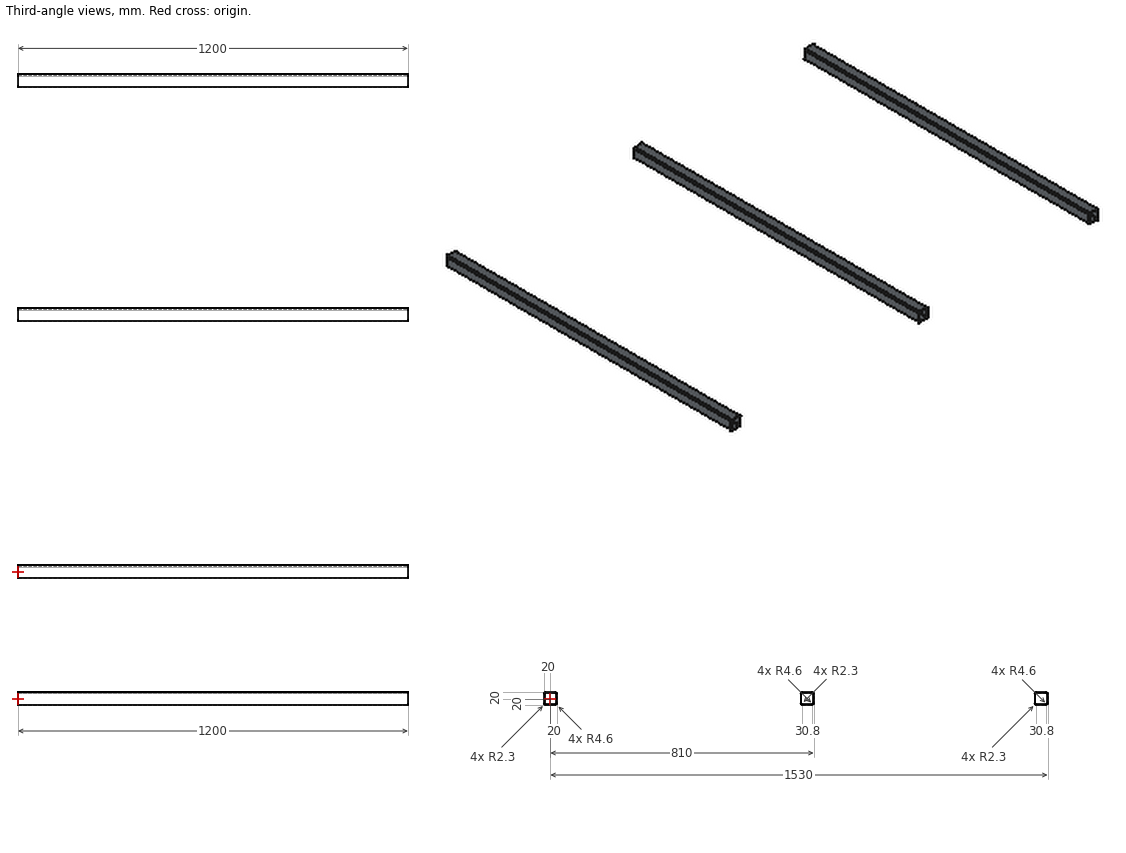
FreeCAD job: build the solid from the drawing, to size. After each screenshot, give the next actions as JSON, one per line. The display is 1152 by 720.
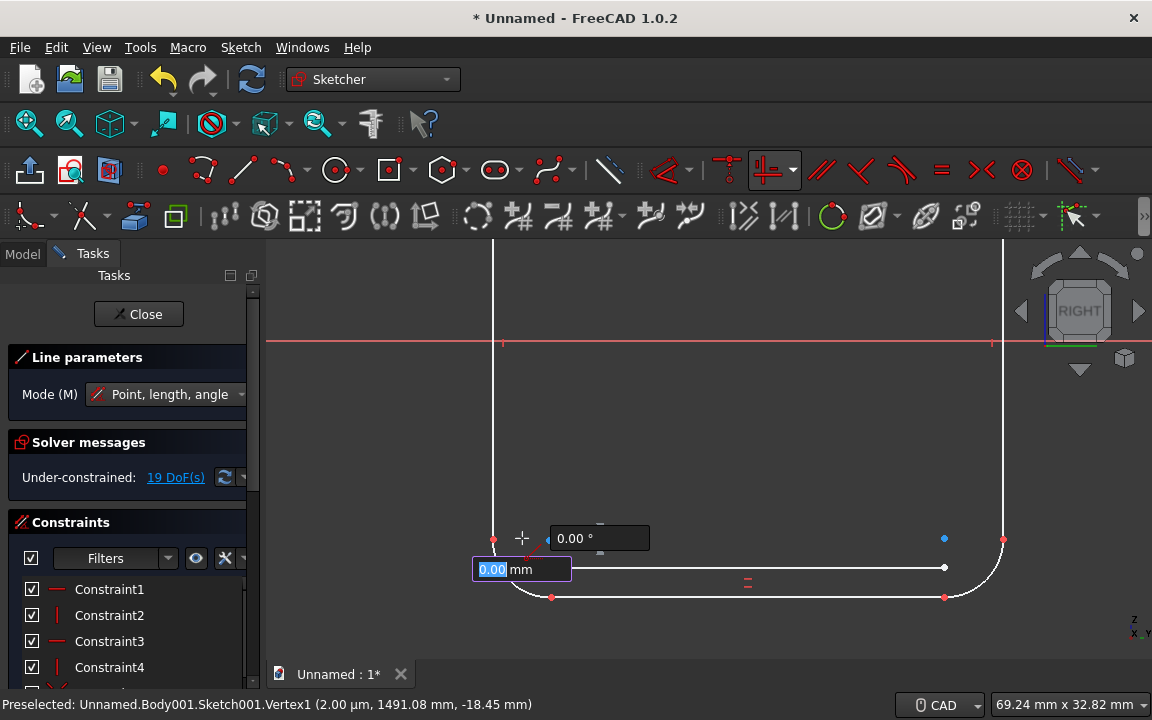
{"action": "scroll", "coordinate": [510, 581], "scroll_direction": "down", "scroll_amount": 3}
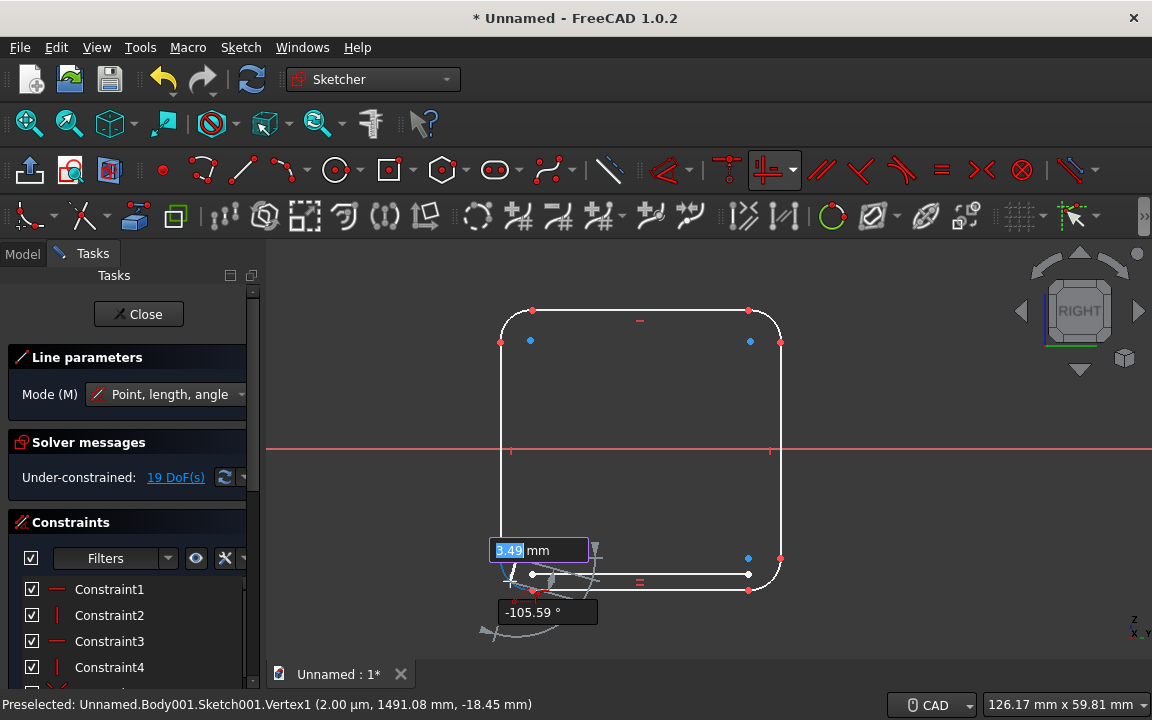
{"action": "left_click", "coordinate": [517, 341]}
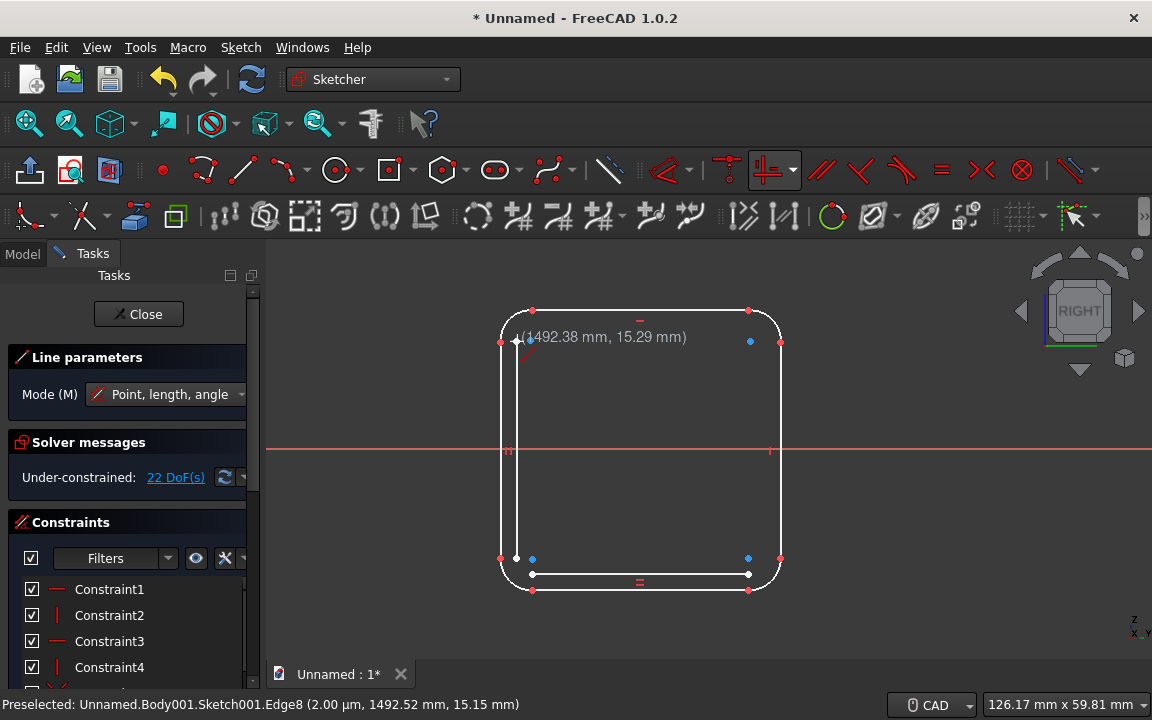
{"action": "left_click", "coordinate": [533, 325]}
{"action": "left_click", "coordinate": [749, 325]}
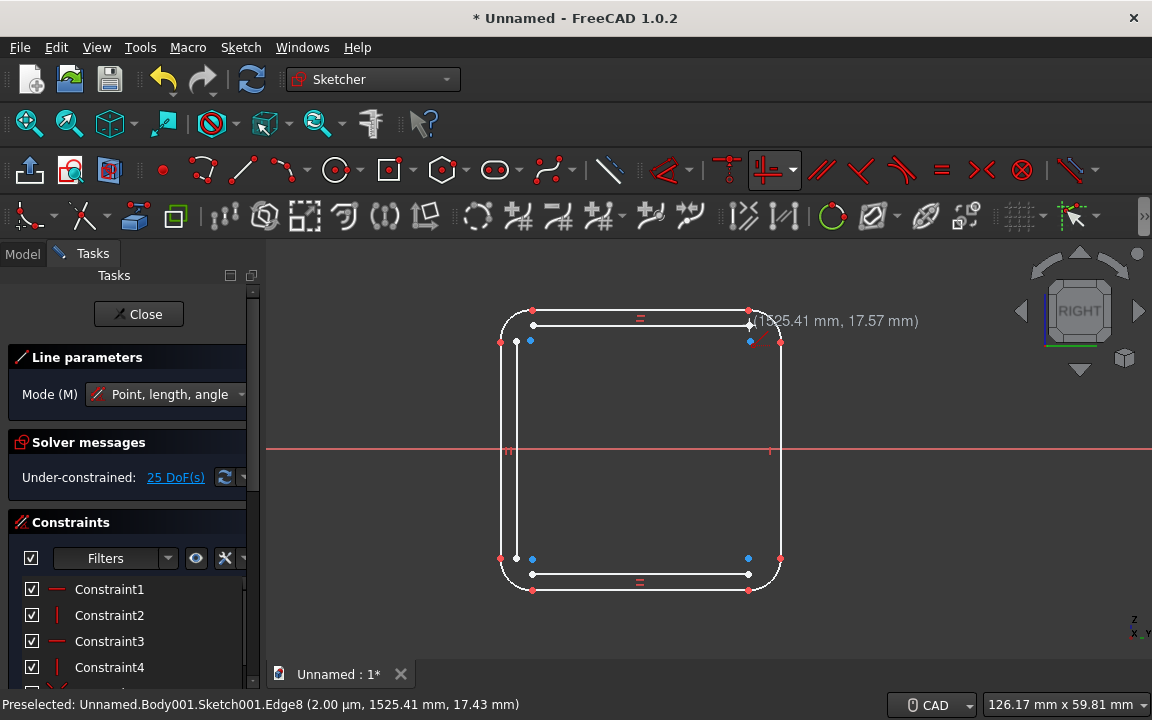
{"action": "left_click", "coordinate": [765, 341]}
{"action": "left_click", "coordinate": [765, 558]}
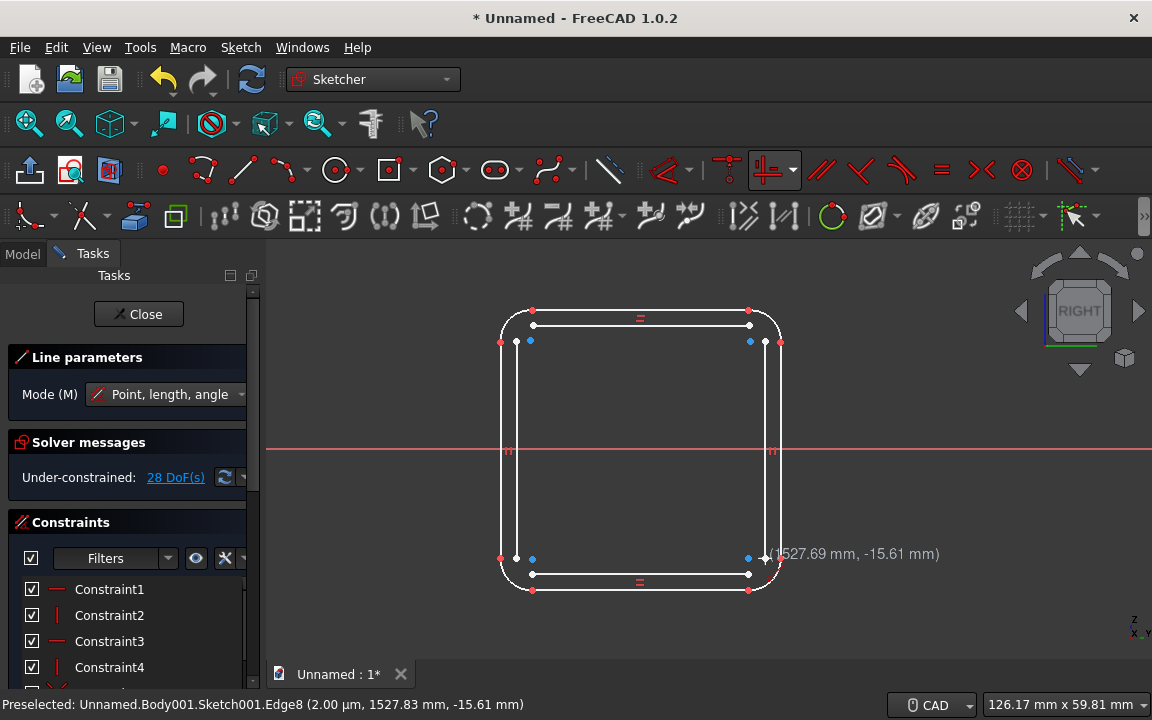
{"action": "left_click", "coordinate": [284, 170]}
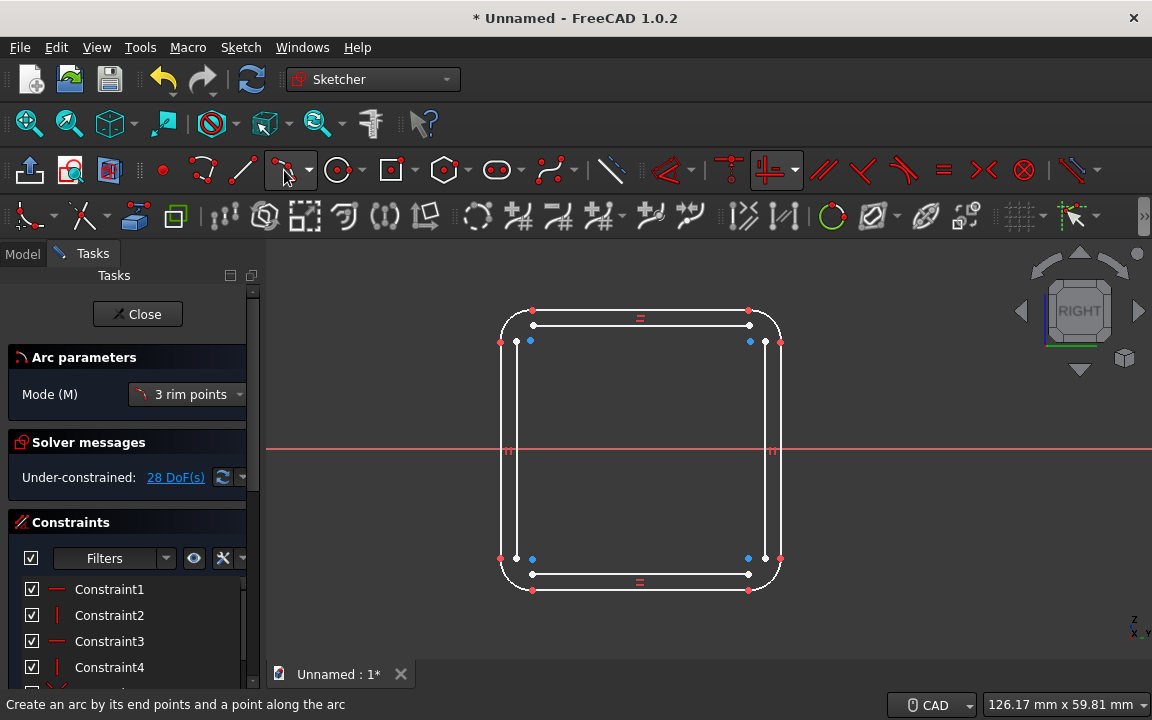
{"action": "left_click", "coordinate": [533, 574]}
{"action": "left_click", "coordinate": [517, 558]}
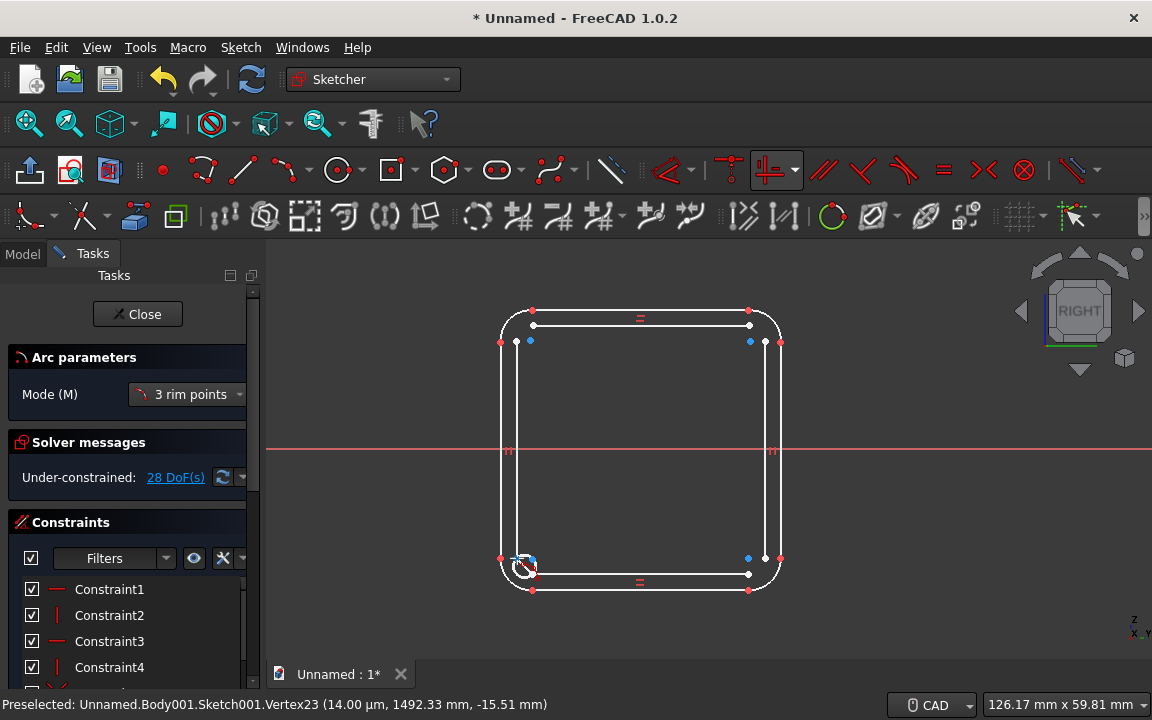
{"action": "scroll", "coordinate": [521, 569], "scroll_direction": "up", "scroll_amount": 7}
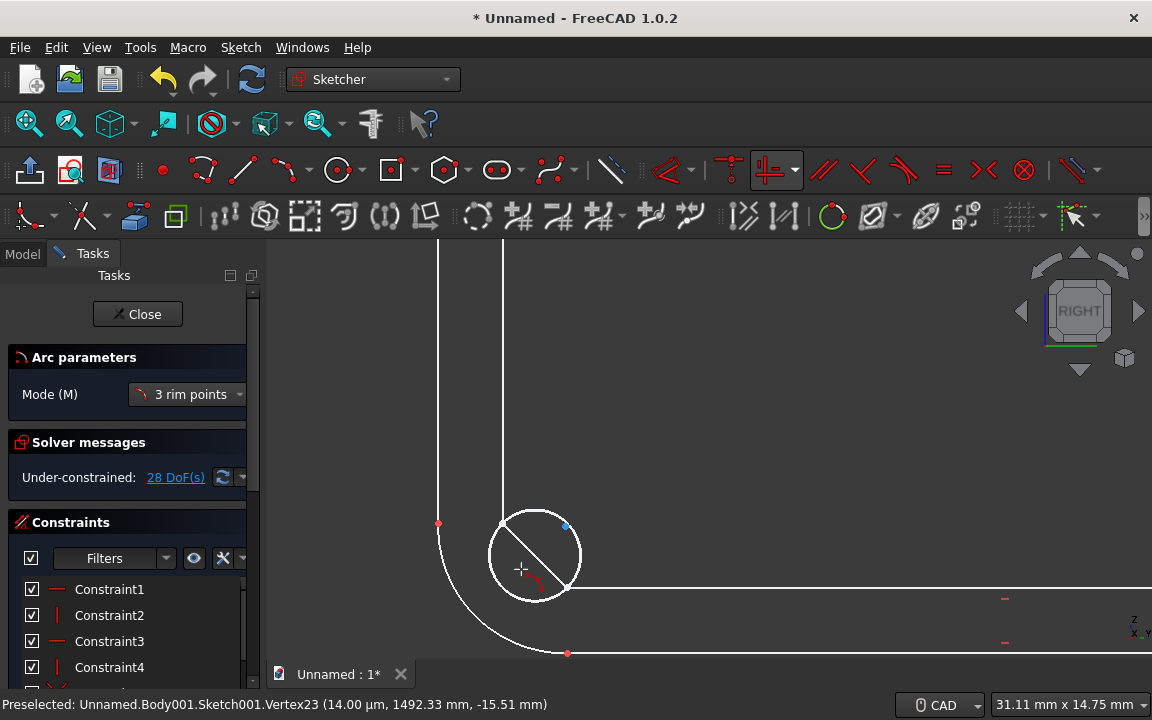
{"action": "left_click", "coordinate": [521, 566]}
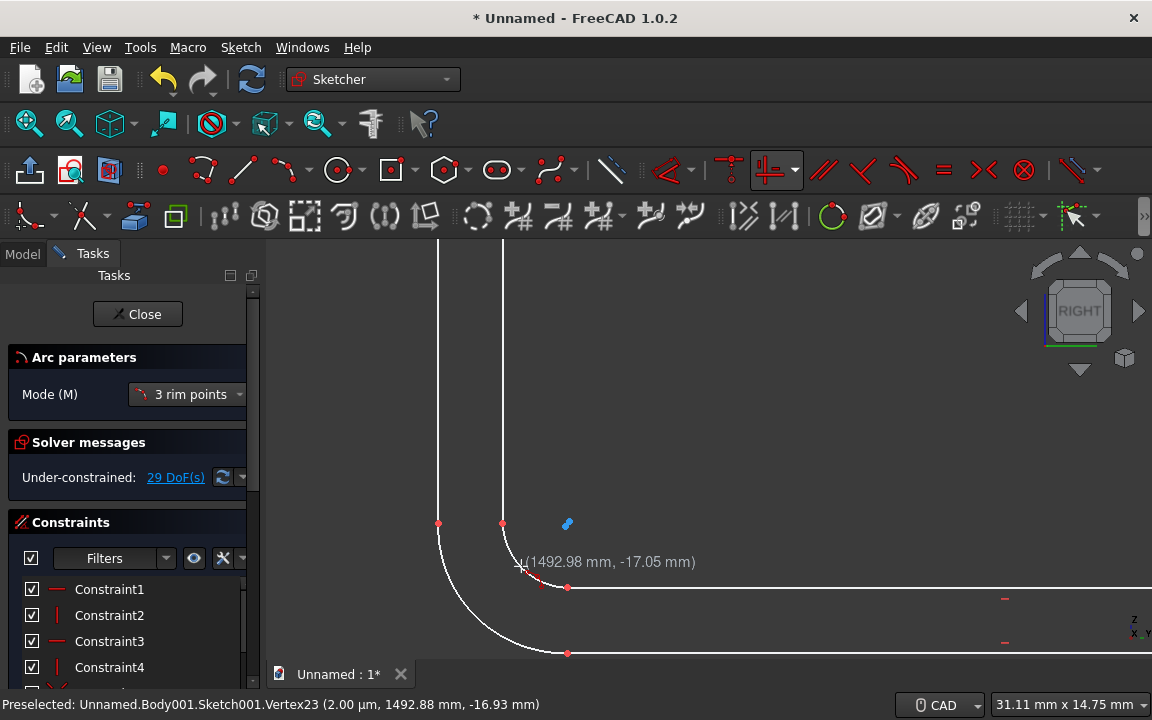
{"action": "scroll", "coordinate": [521, 569], "scroll_direction": "down", "scroll_amount": 7}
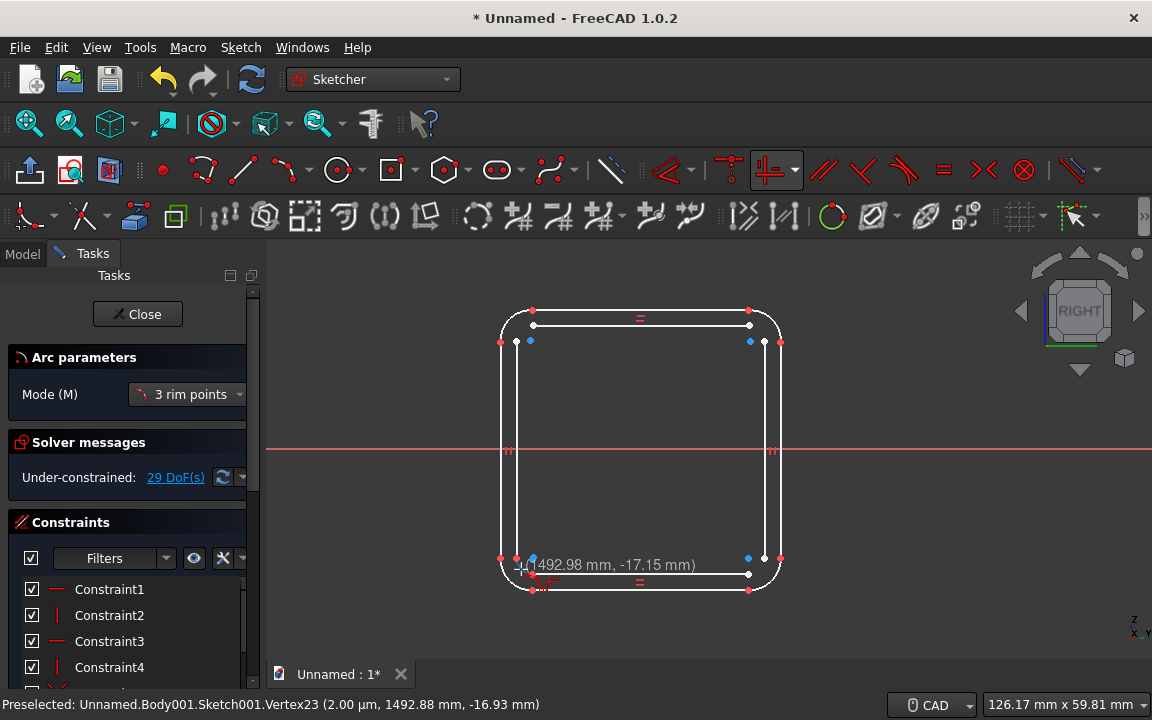
{"action": "left_click", "coordinate": [517, 342]}
{"action": "left_click", "coordinate": [533, 326]}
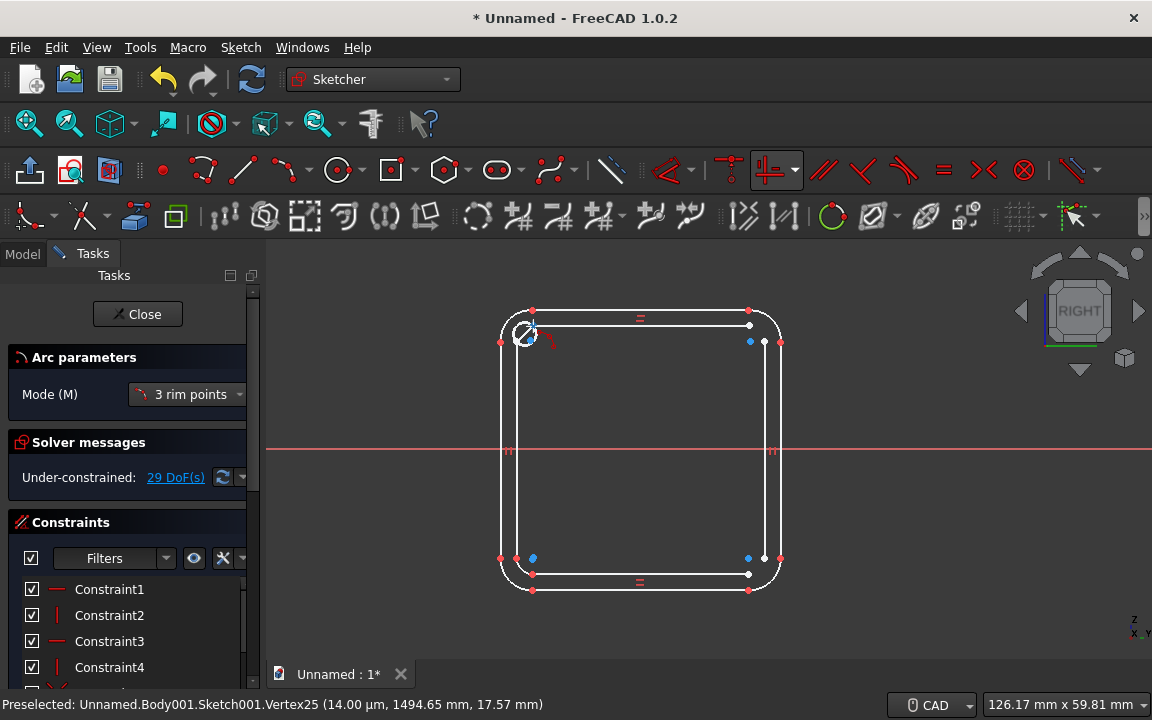
{"action": "scroll", "coordinate": [521, 330], "scroll_direction": "up", "scroll_amount": 7}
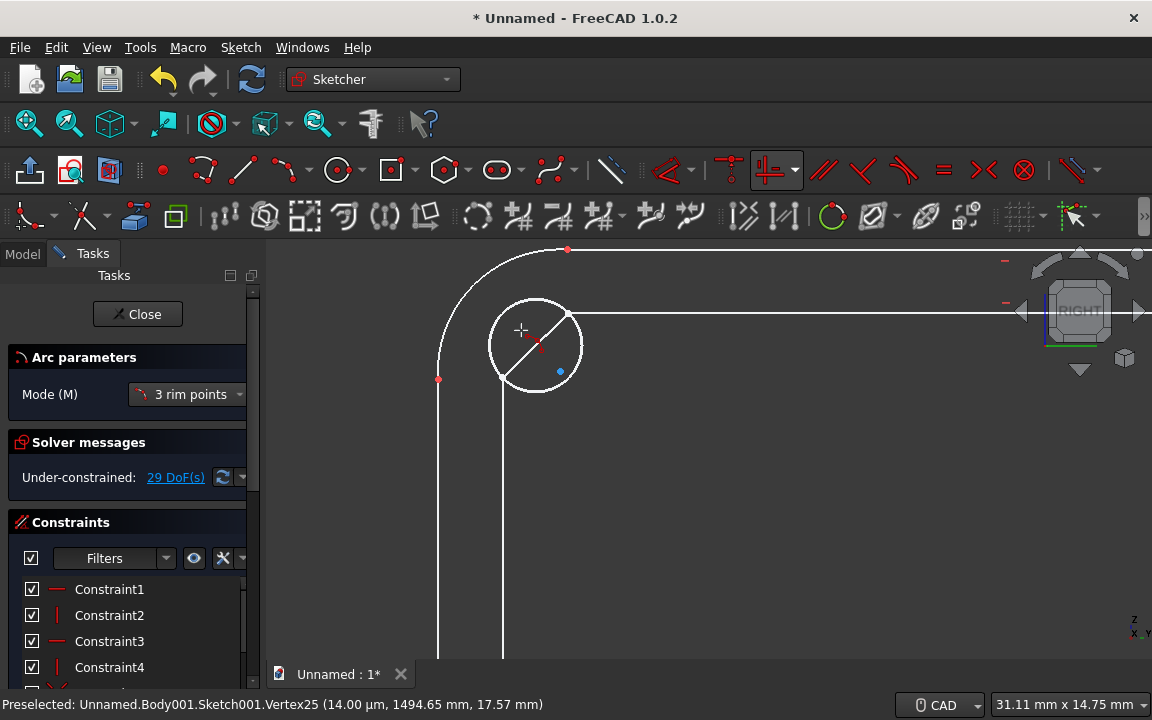
{"action": "left_click", "coordinate": [521, 329]}